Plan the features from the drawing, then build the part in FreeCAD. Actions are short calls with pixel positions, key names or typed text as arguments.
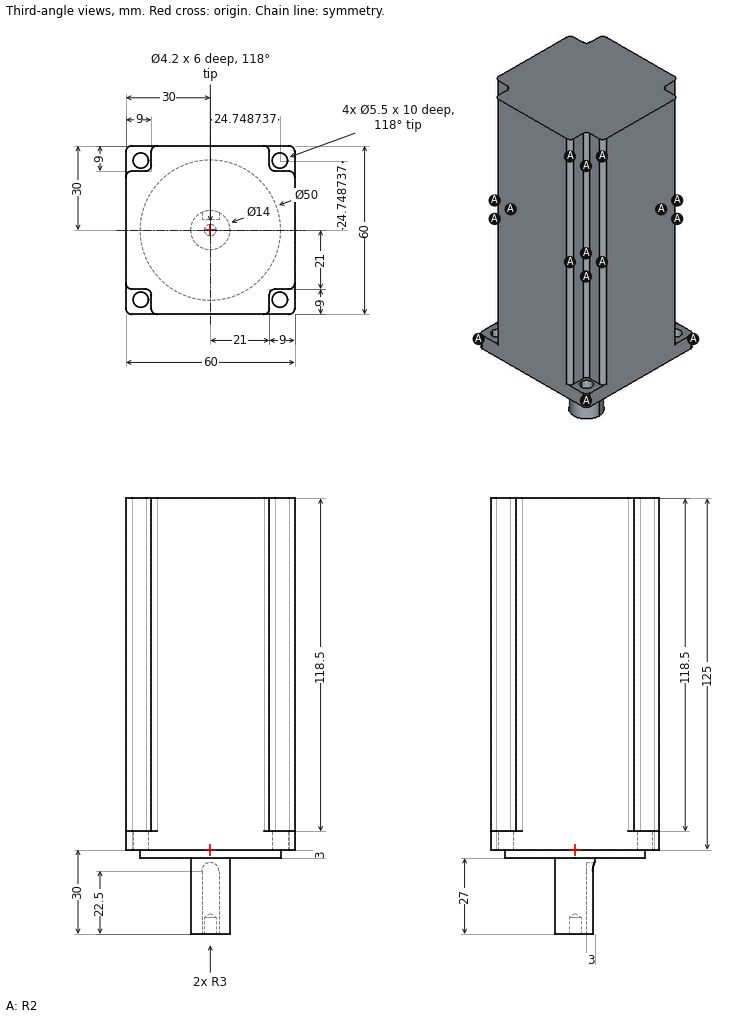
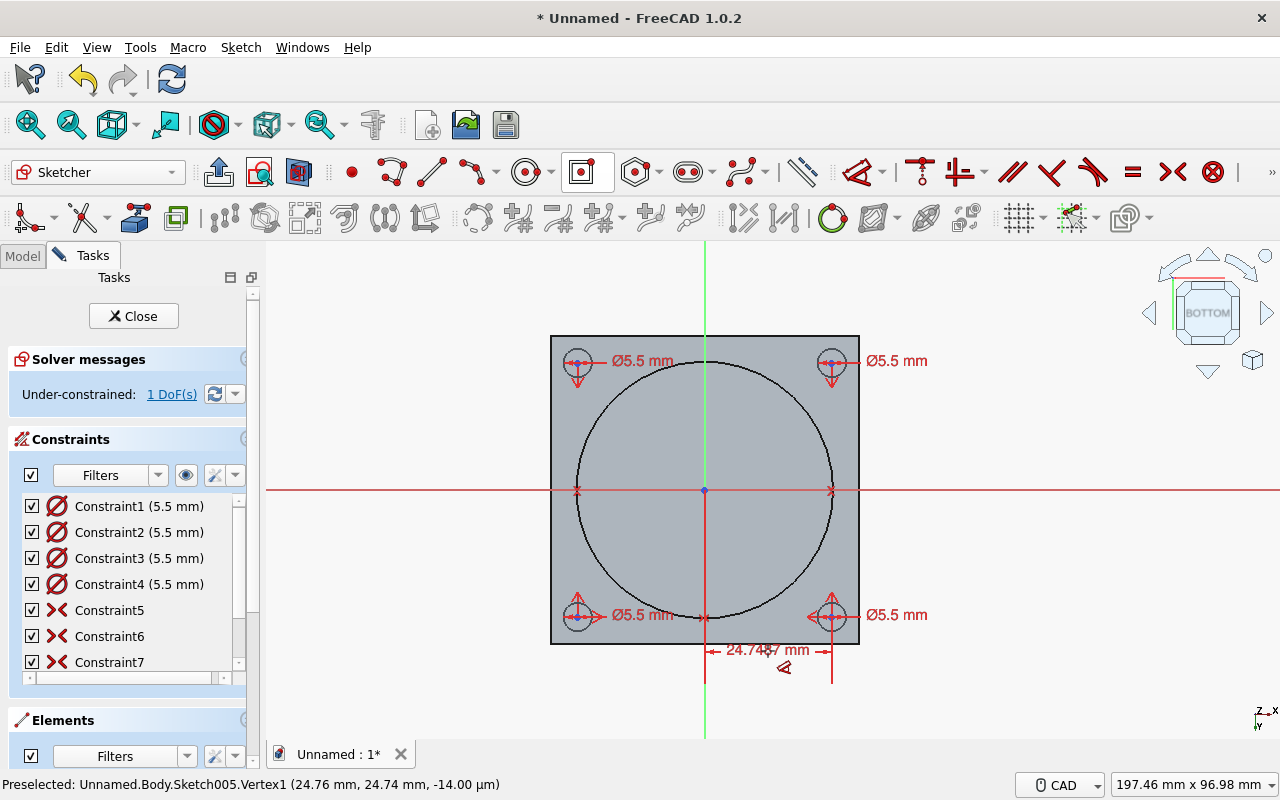
click(832, 617)
click(866, 554)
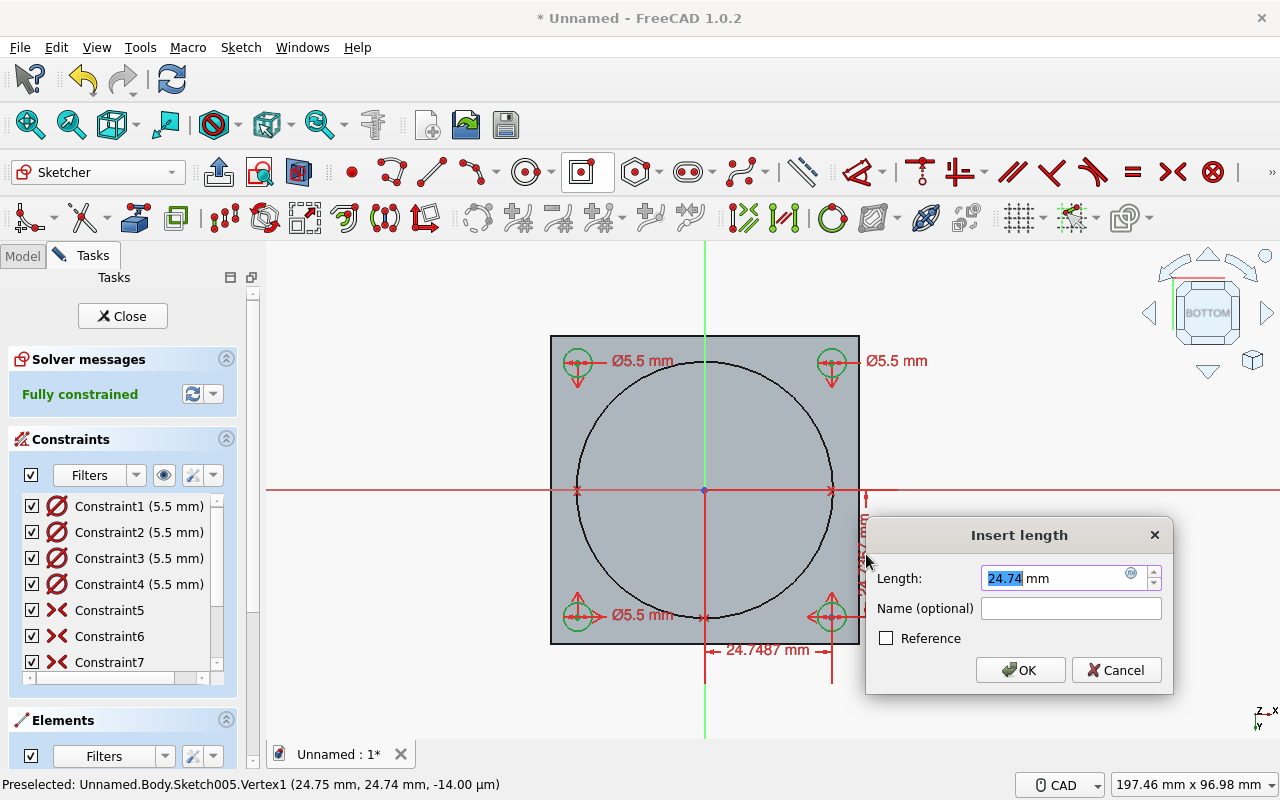
text(24.748737)
key(Return)
key(Escape)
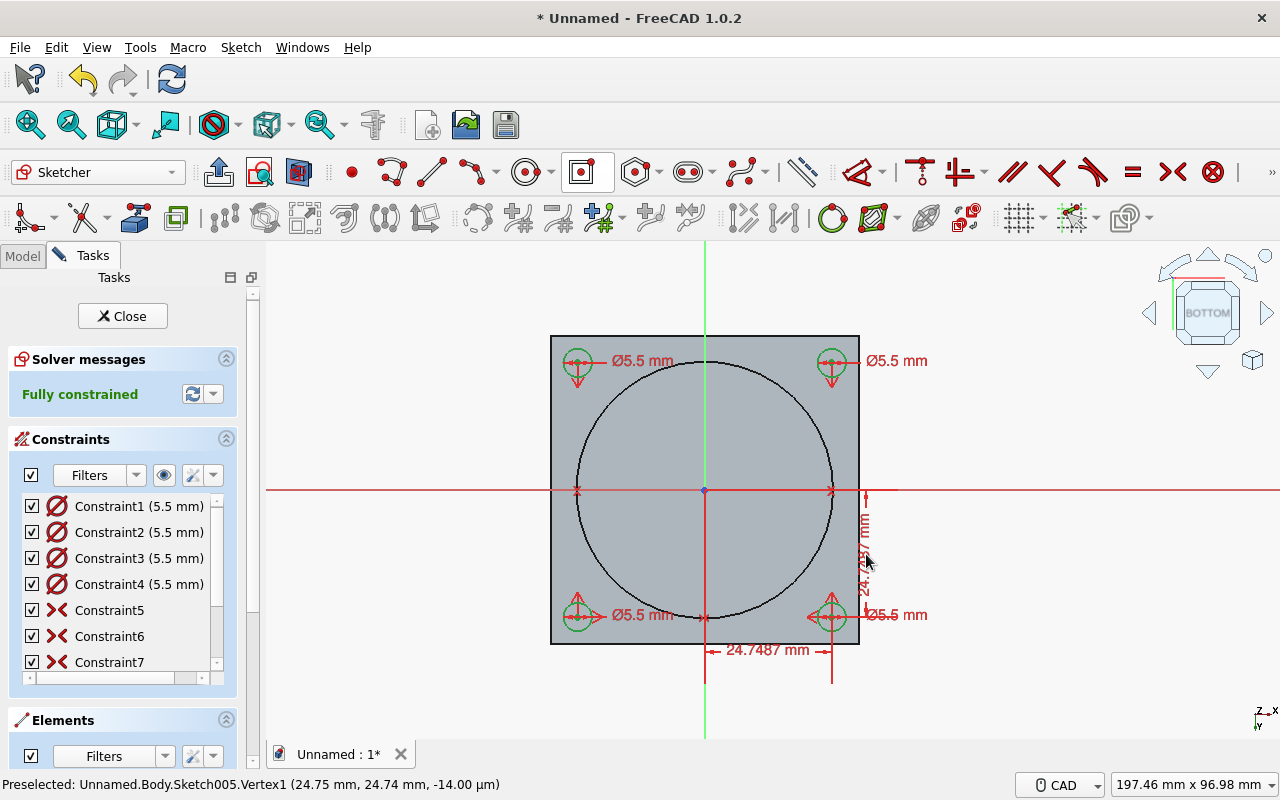
click(123, 316)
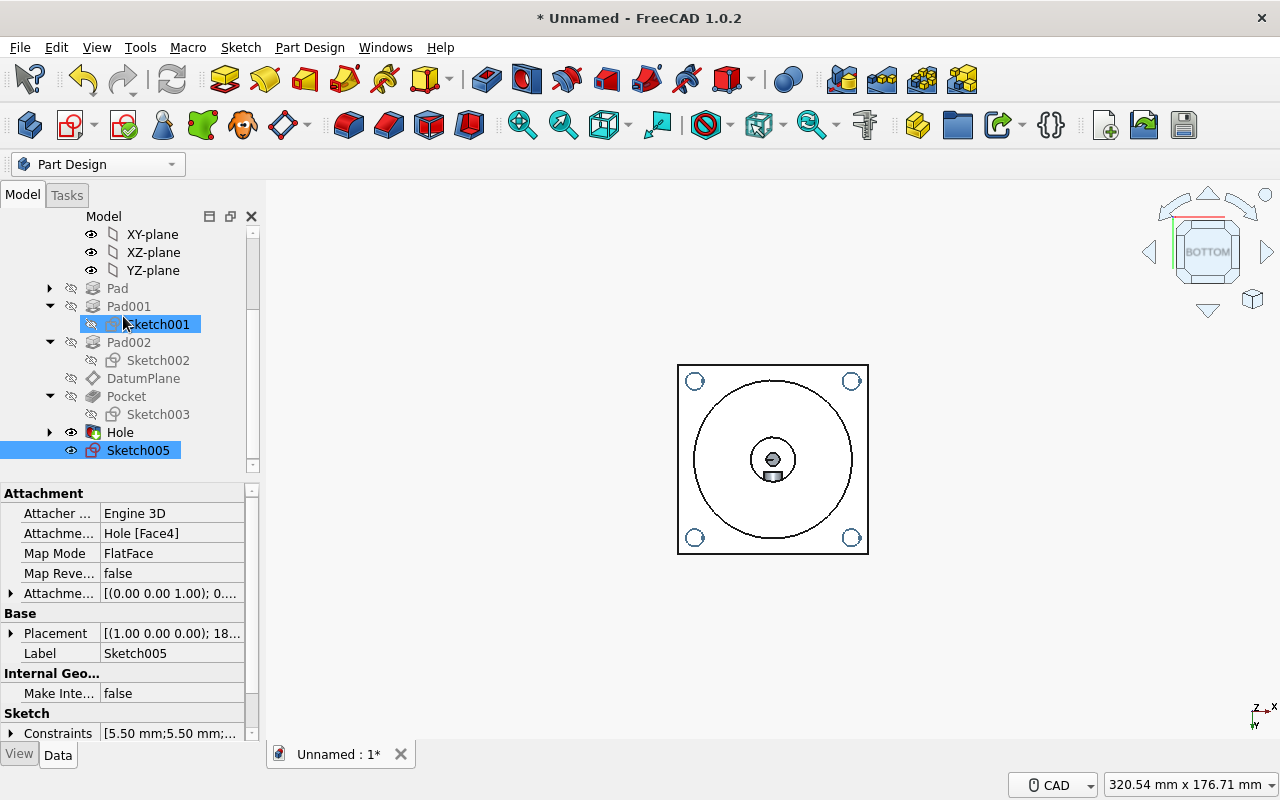
click(528, 80)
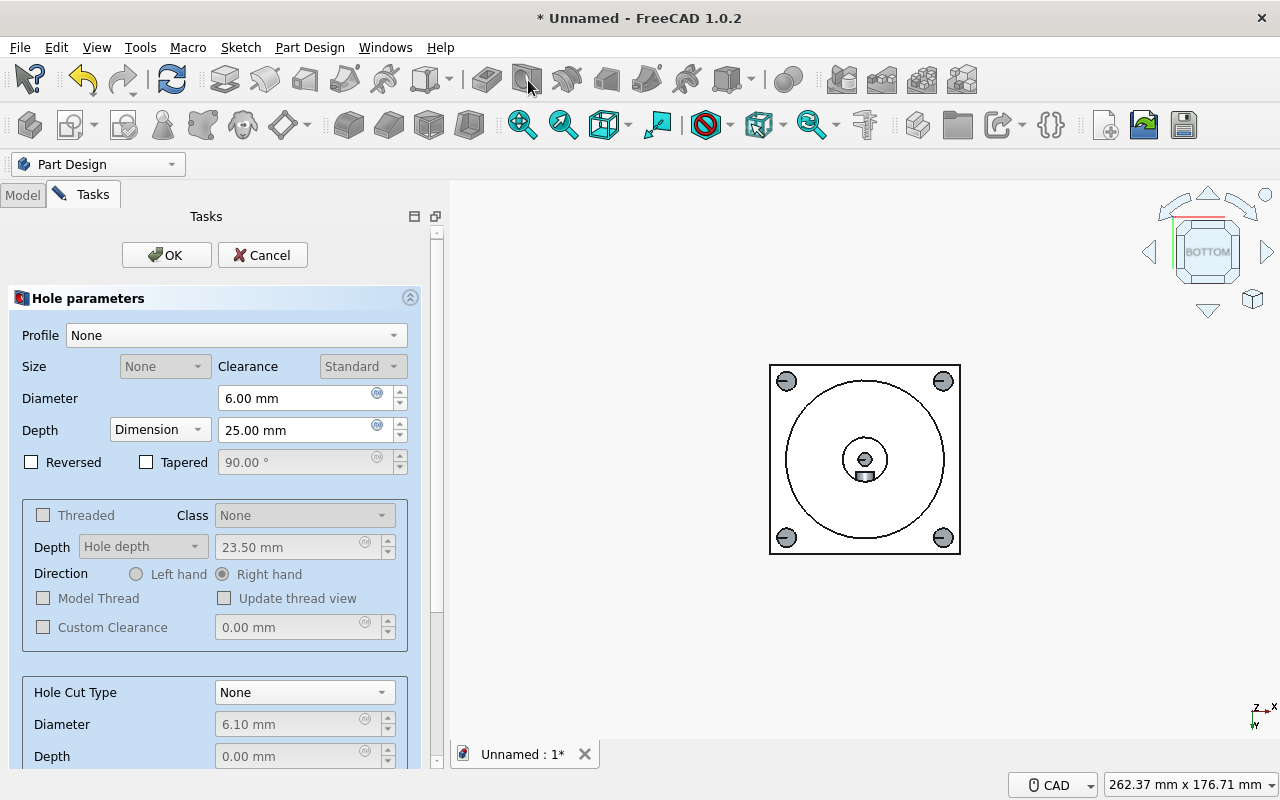
triple_click(305, 398)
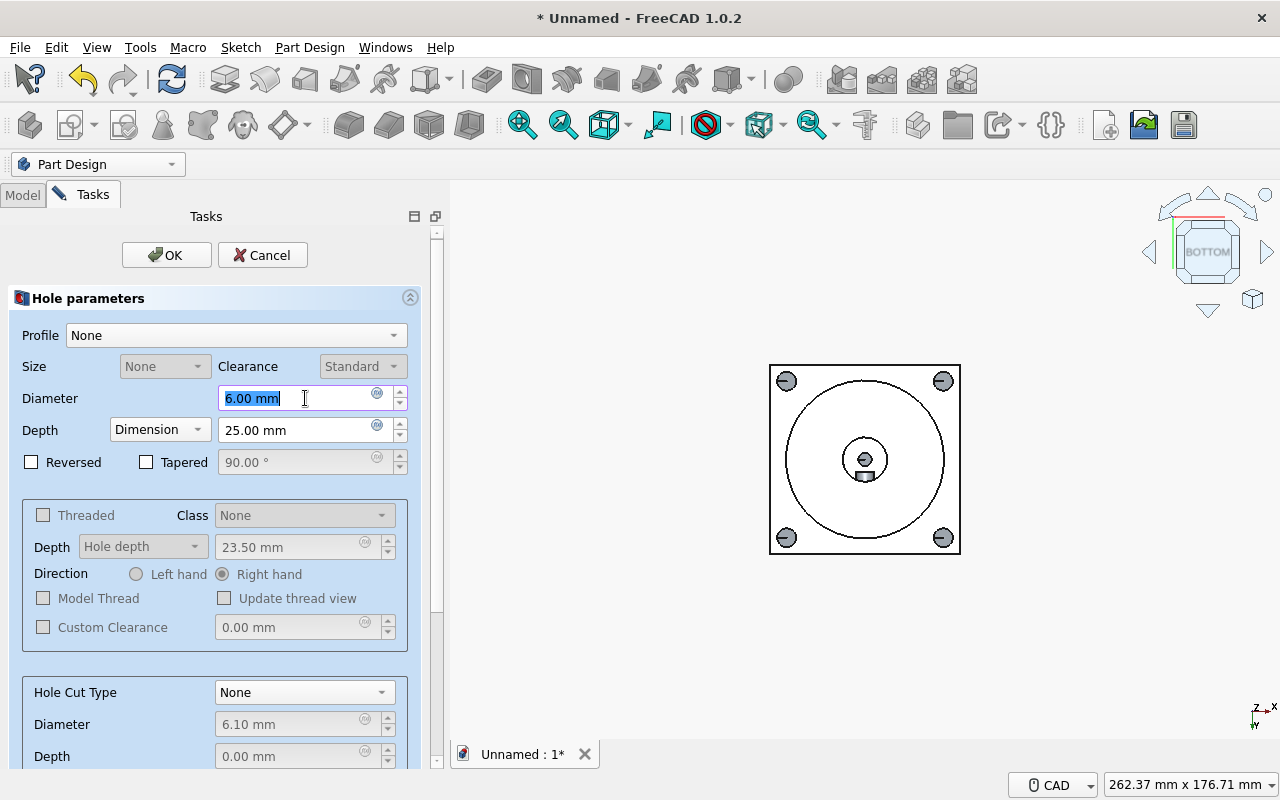
text(5.5)
key(Tab)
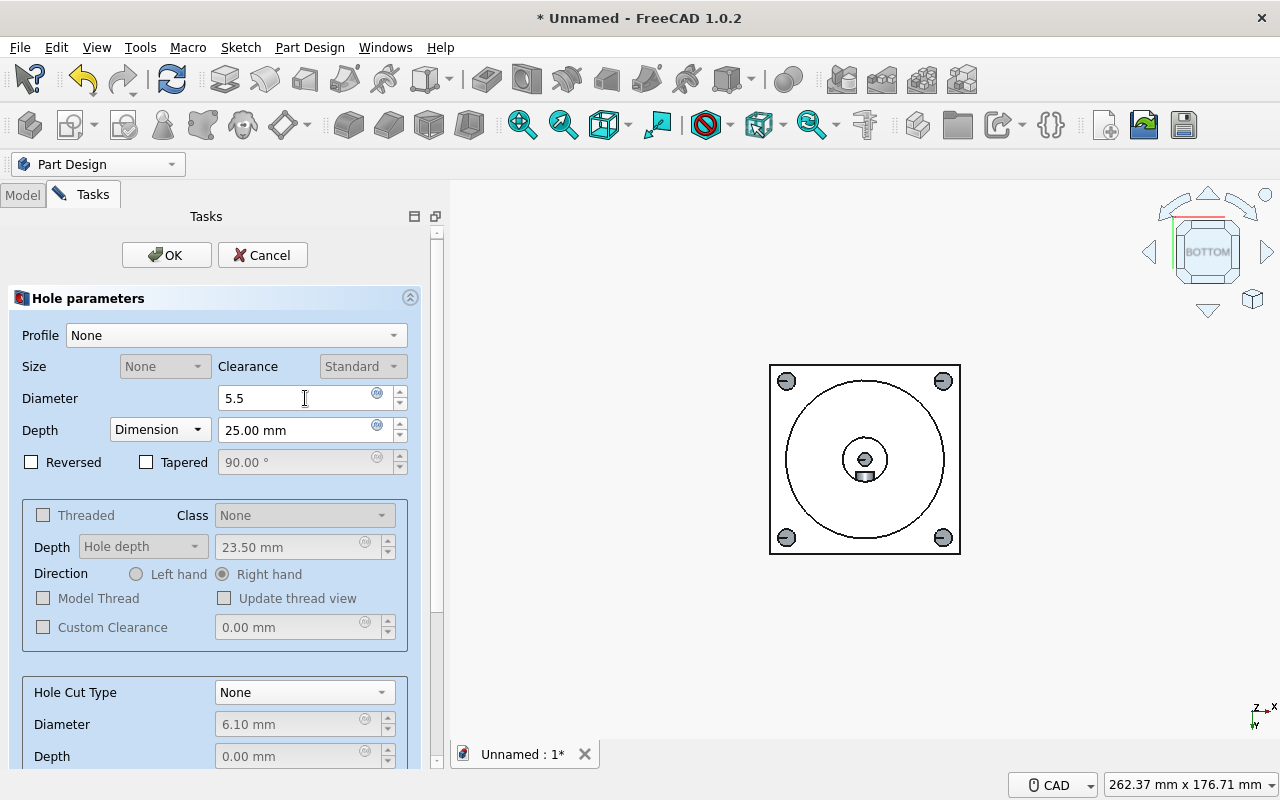
triple_click(305, 430)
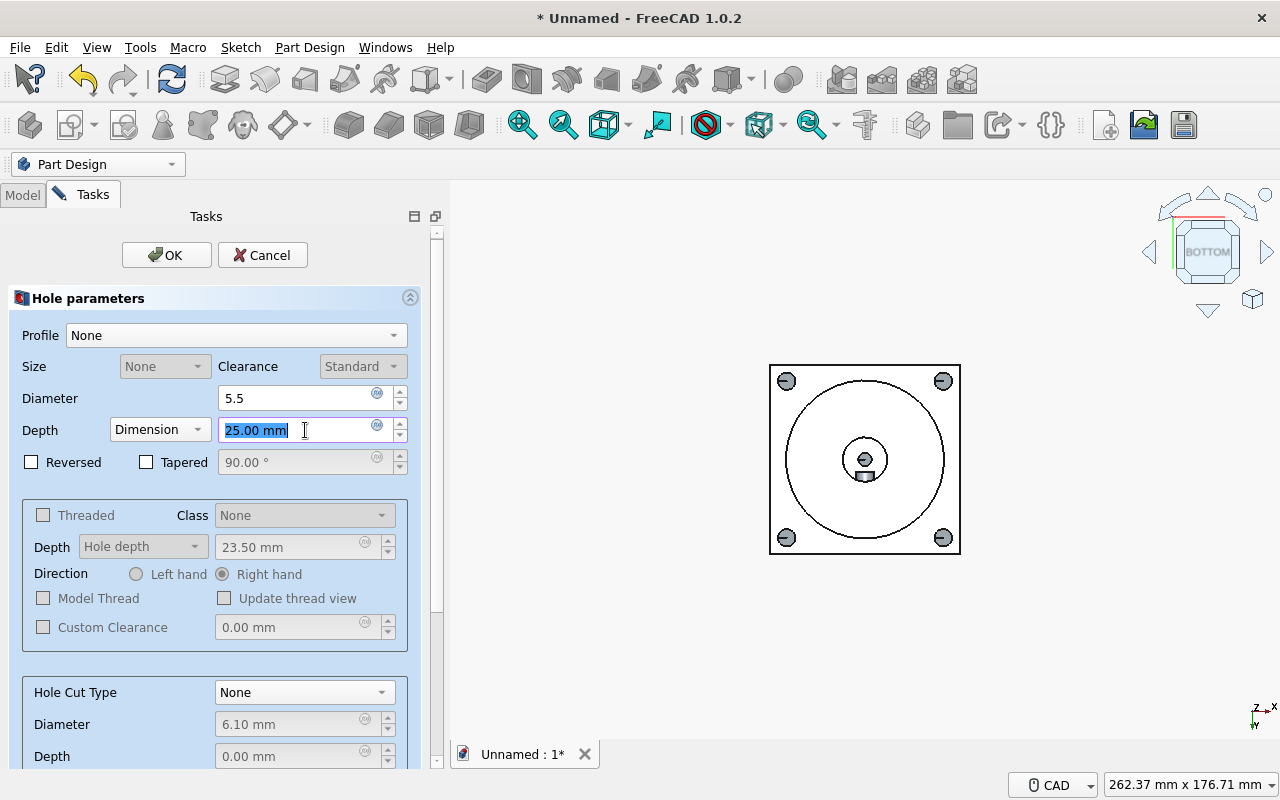
text(10)
key(Tab)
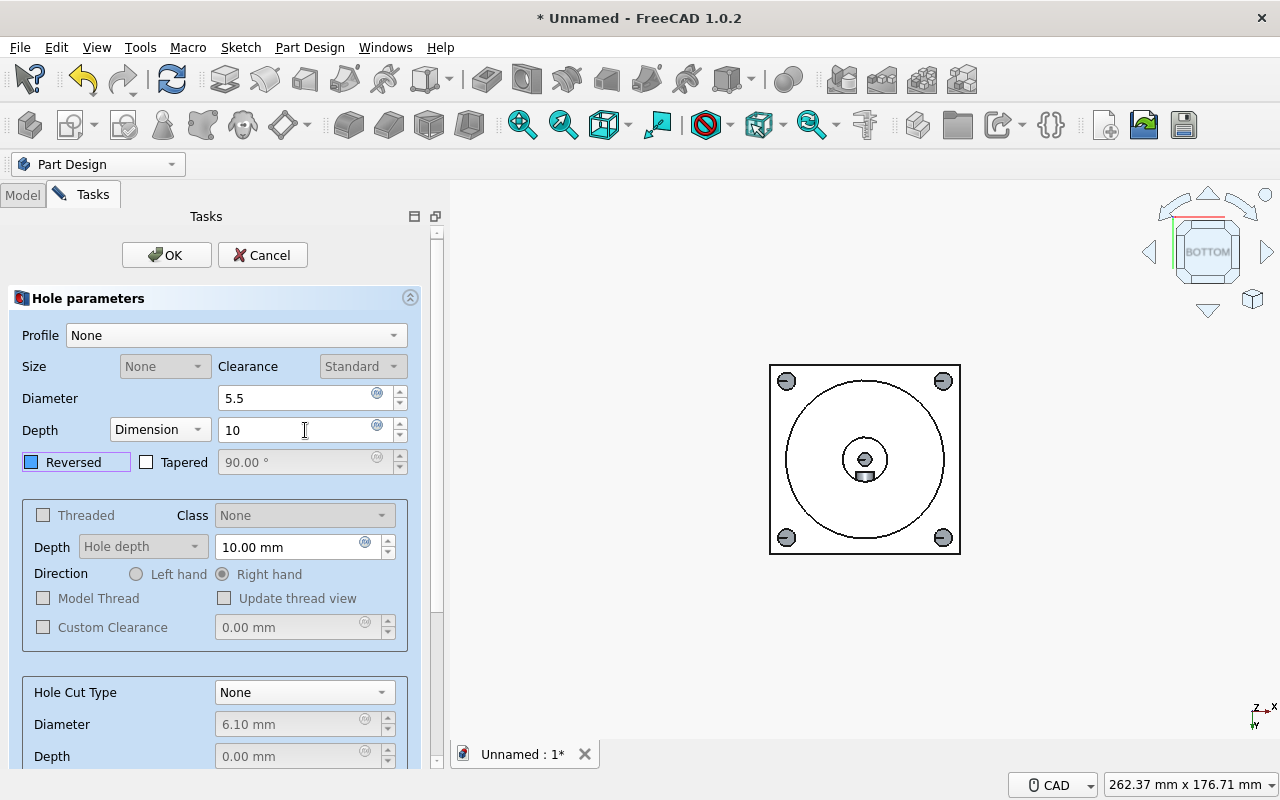
click(167, 255)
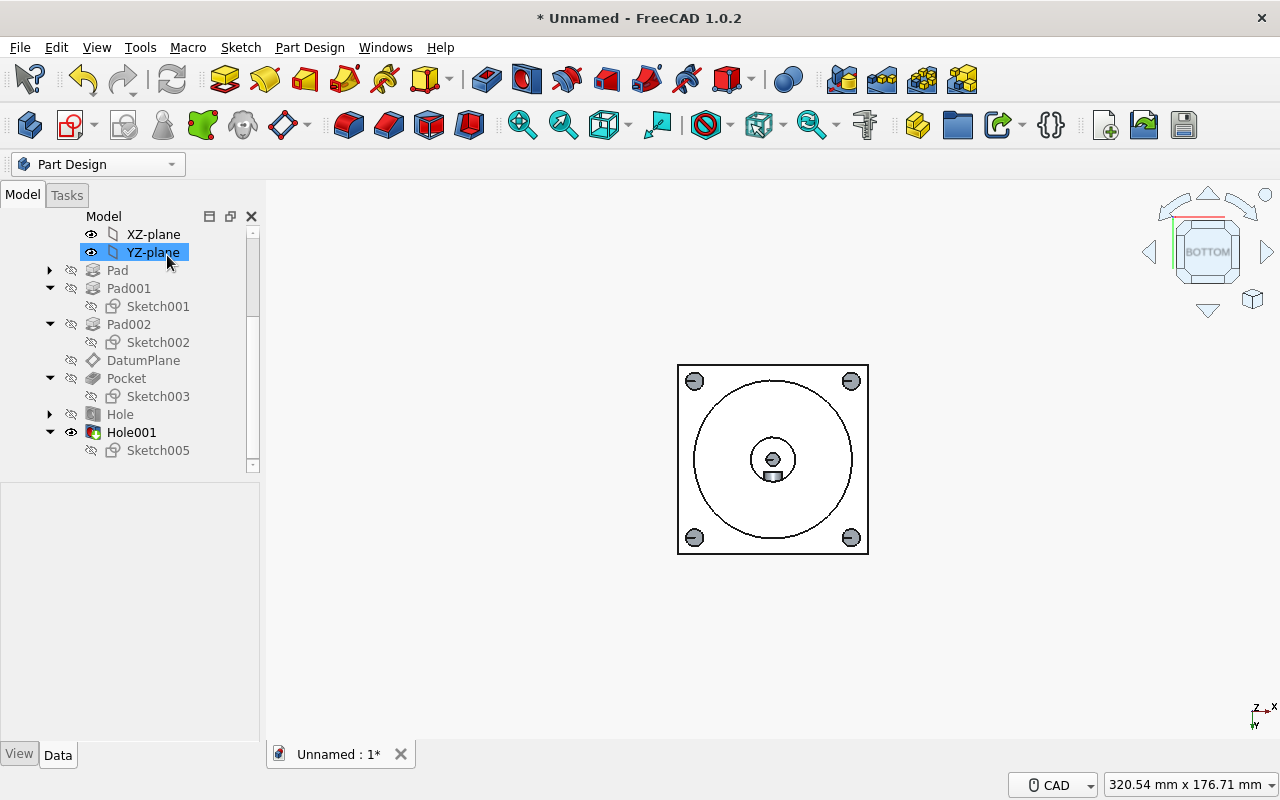
click(524, 126)